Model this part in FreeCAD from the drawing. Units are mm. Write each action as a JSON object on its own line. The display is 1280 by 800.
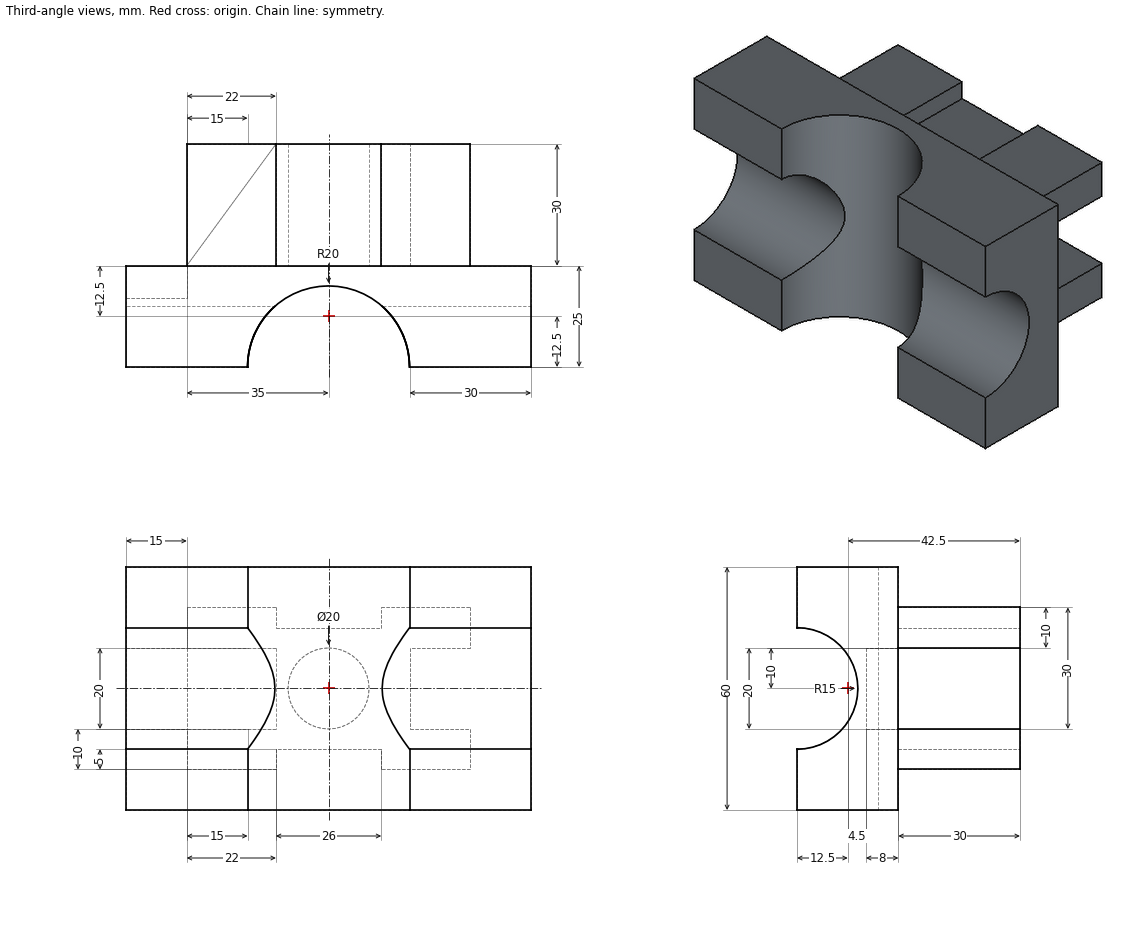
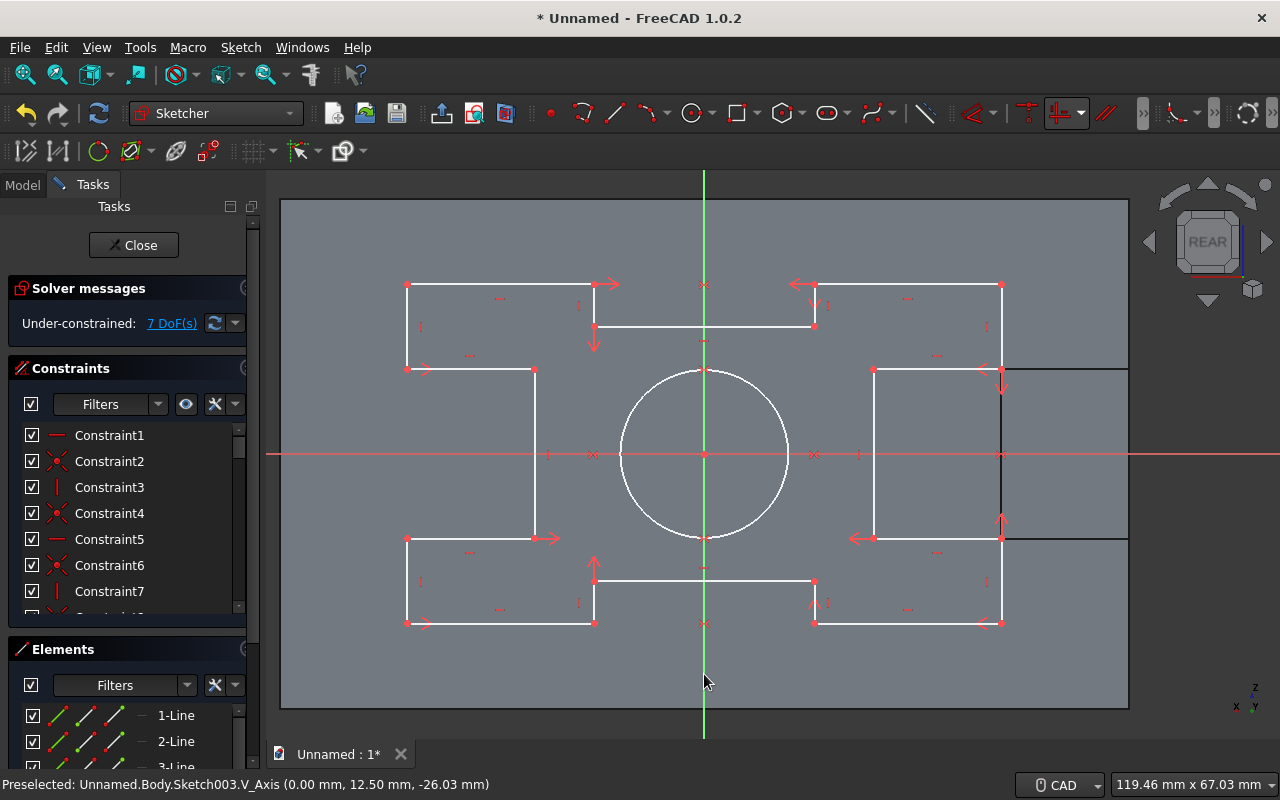
{"action": "left_click", "coordinate": [972, 114]}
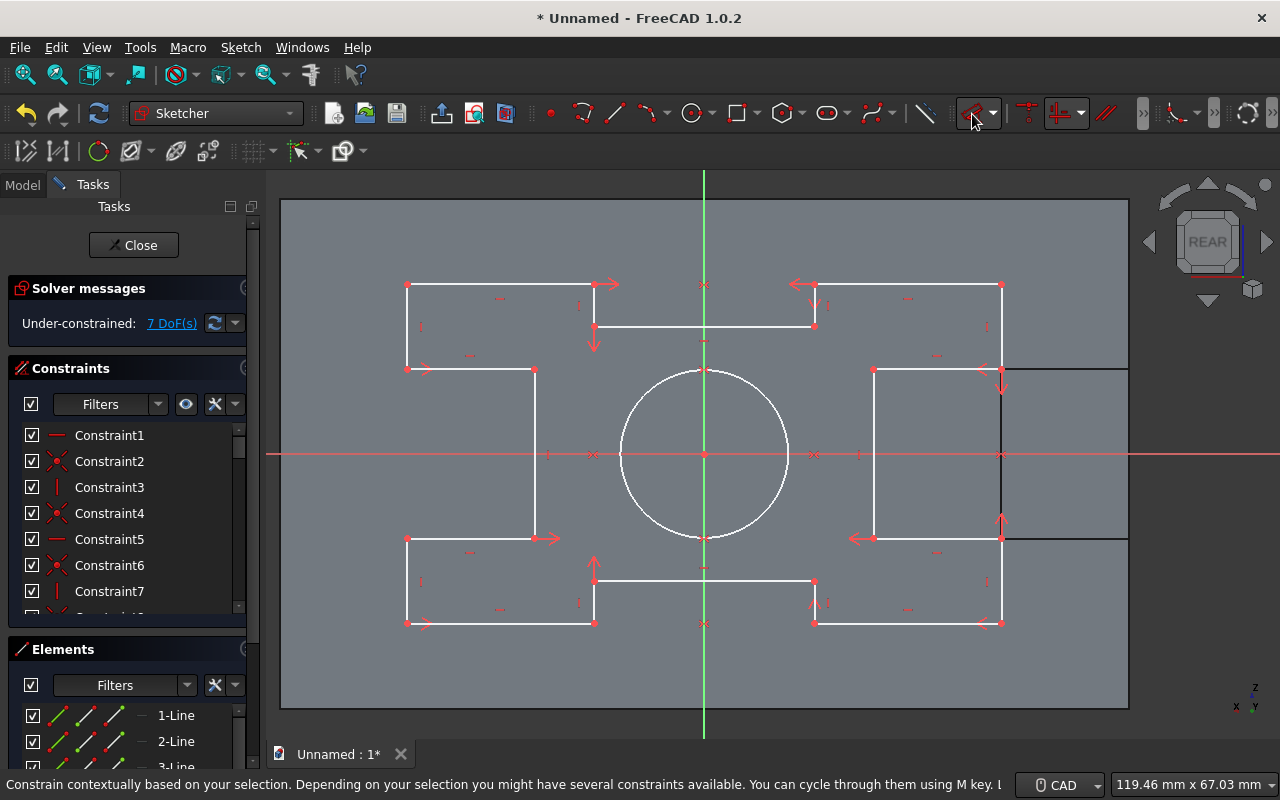
{"action": "left_click", "coordinate": [763, 394]}
{"action": "left_click", "coordinate": [785, 371]}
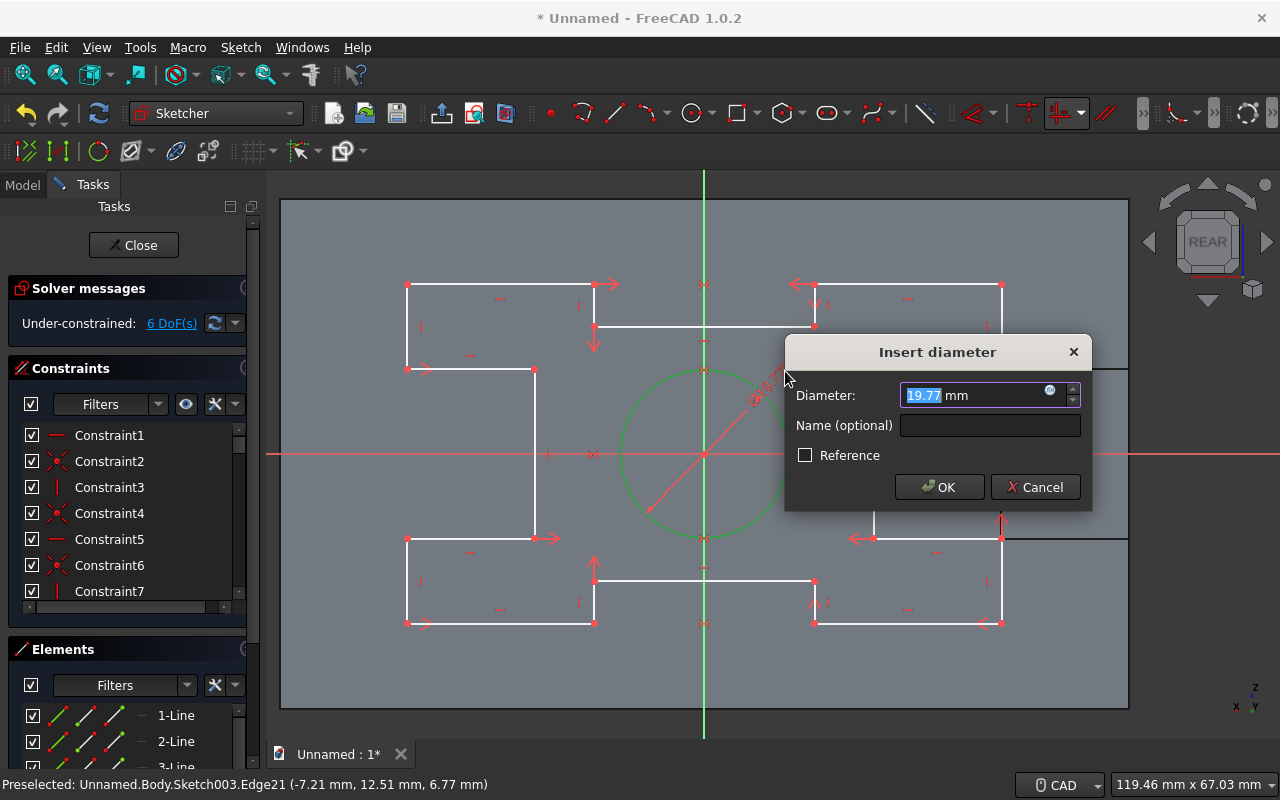
{"action": "type", "text": "20"}
{"action": "key", "text": "Return"}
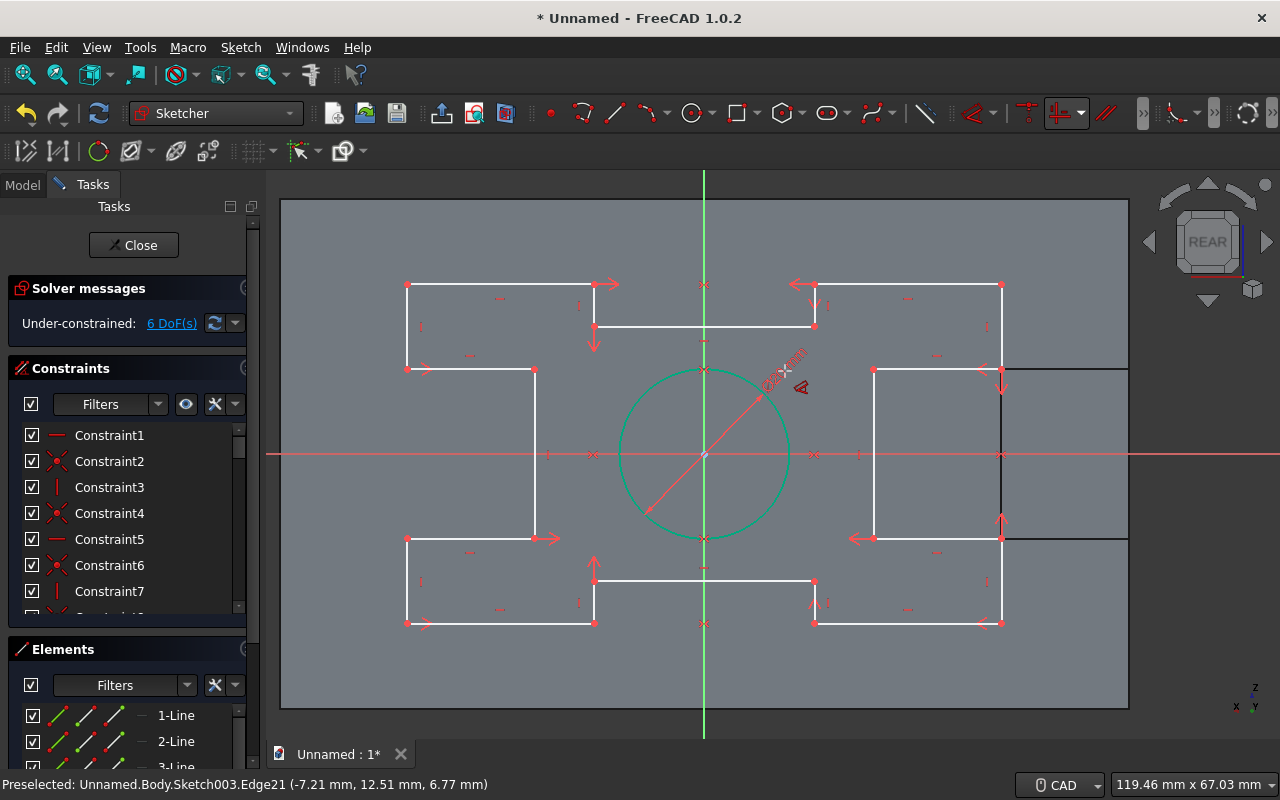
{"action": "left_click", "coordinate": [815, 594]}
{"action": "left_click", "coordinate": [849, 603]}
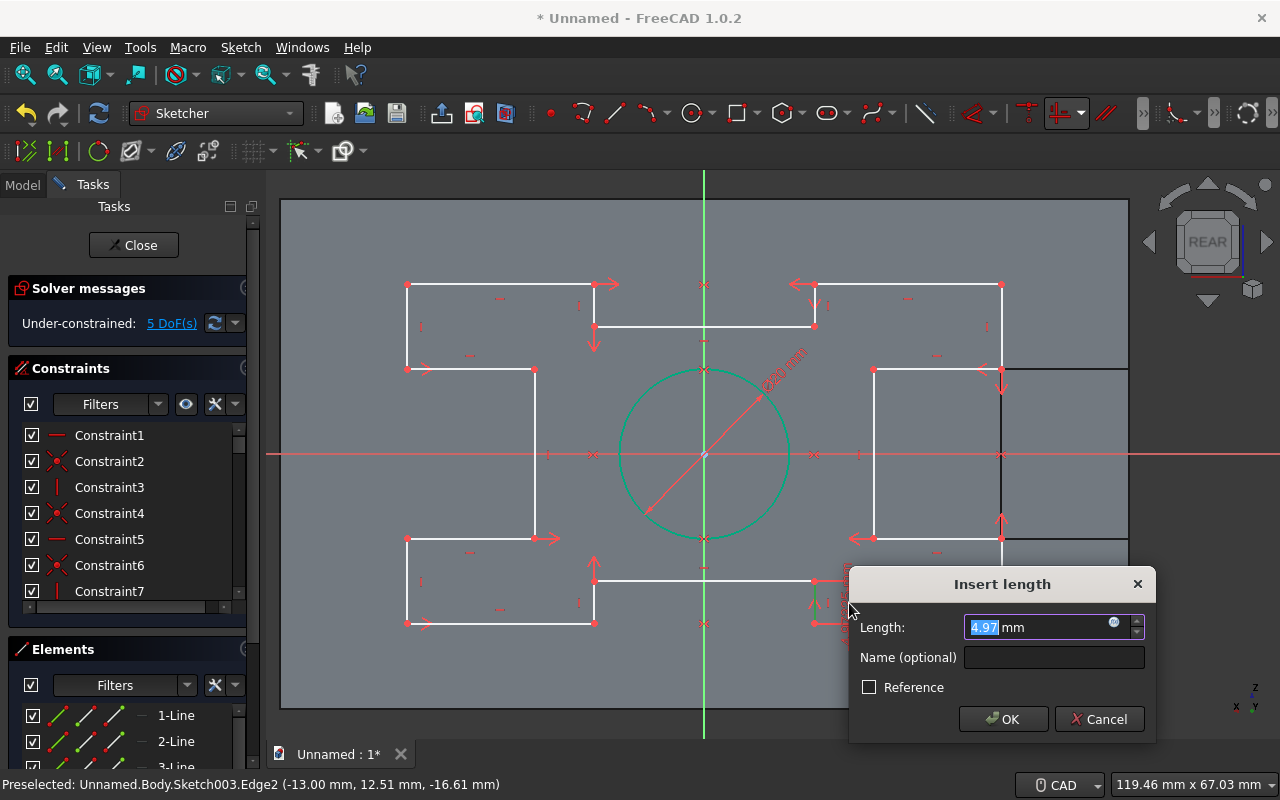
{"action": "type", "text": "5"}
{"action": "key", "text": "Return"}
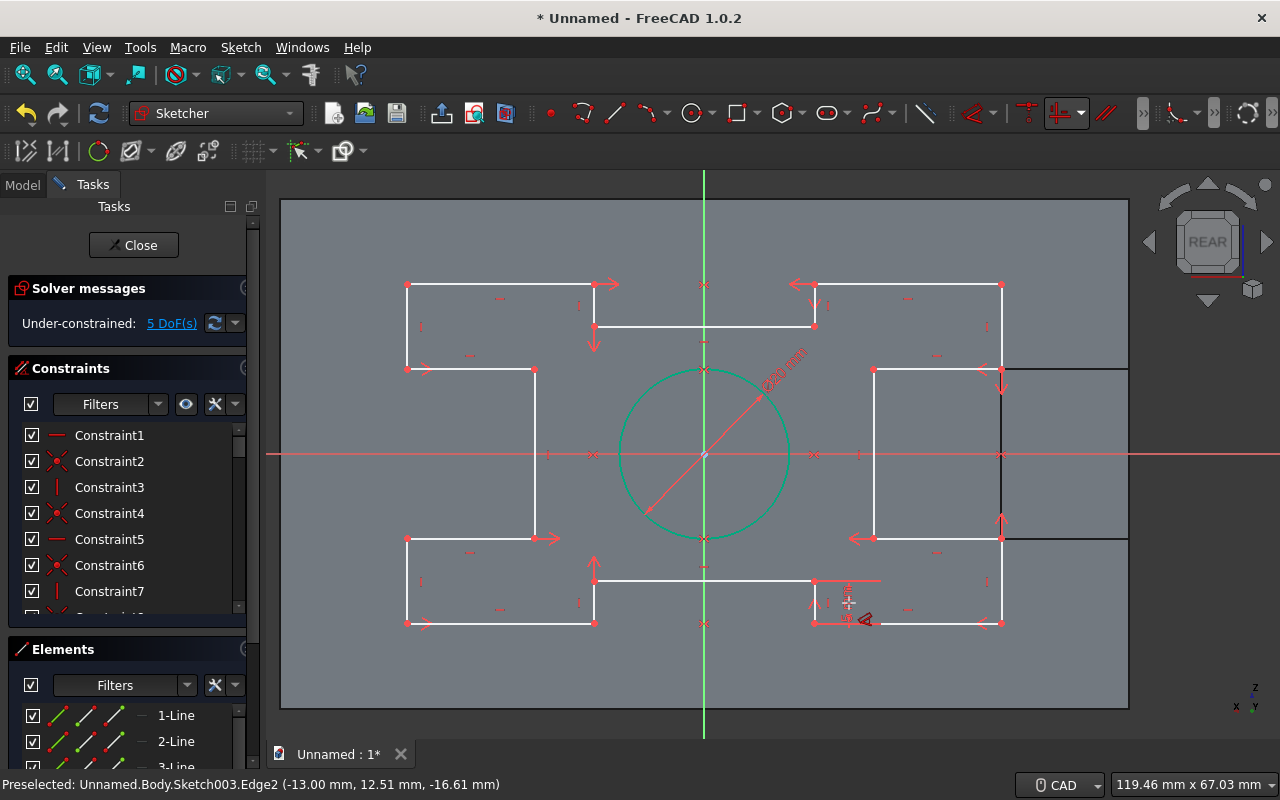
{"action": "left_click", "coordinate": [660, 581]}
{"action": "left_click", "coordinate": [654, 615]}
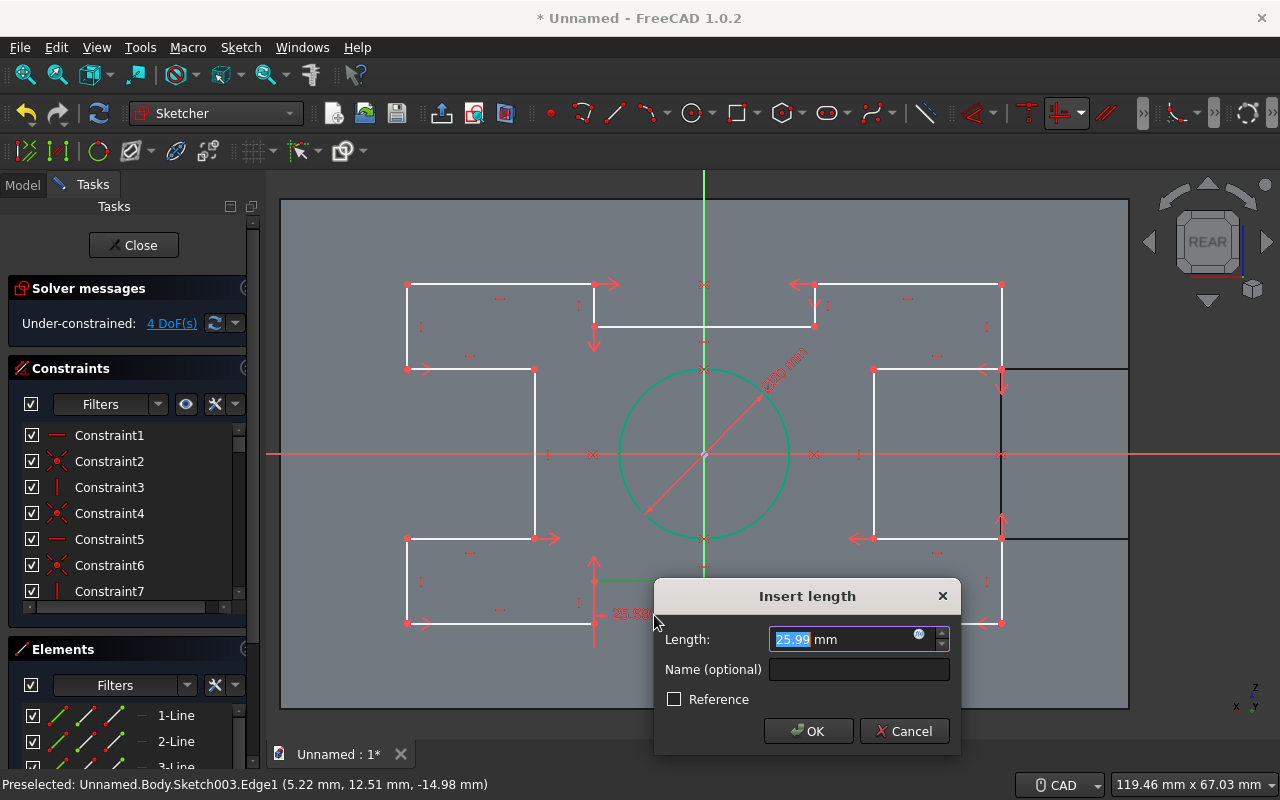
{"action": "type", "text": "26"}
{"action": "key", "text": "Return"}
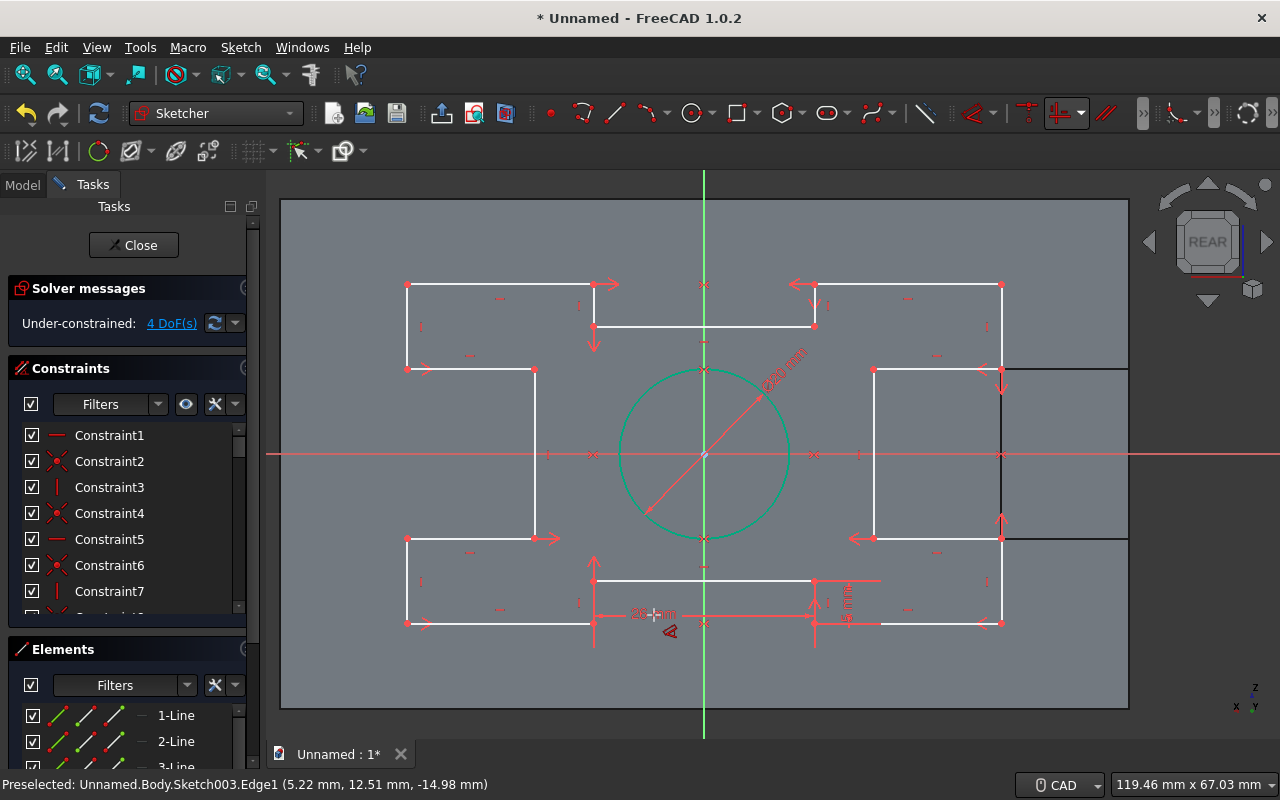
{"action": "left_click", "coordinate": [871, 624]}
{"action": "left_click", "coordinate": [908, 658]}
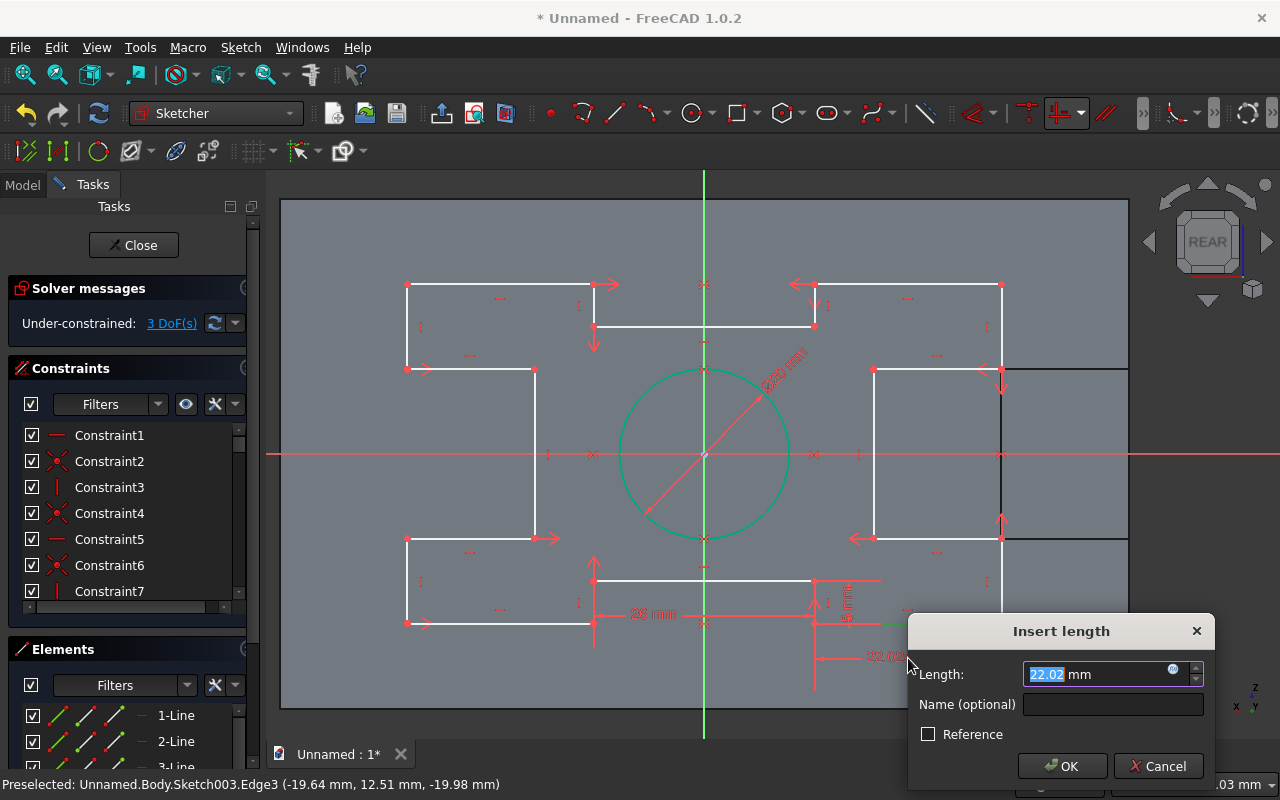
{"action": "type", "text": "22"}
{"action": "key", "text": "Return"}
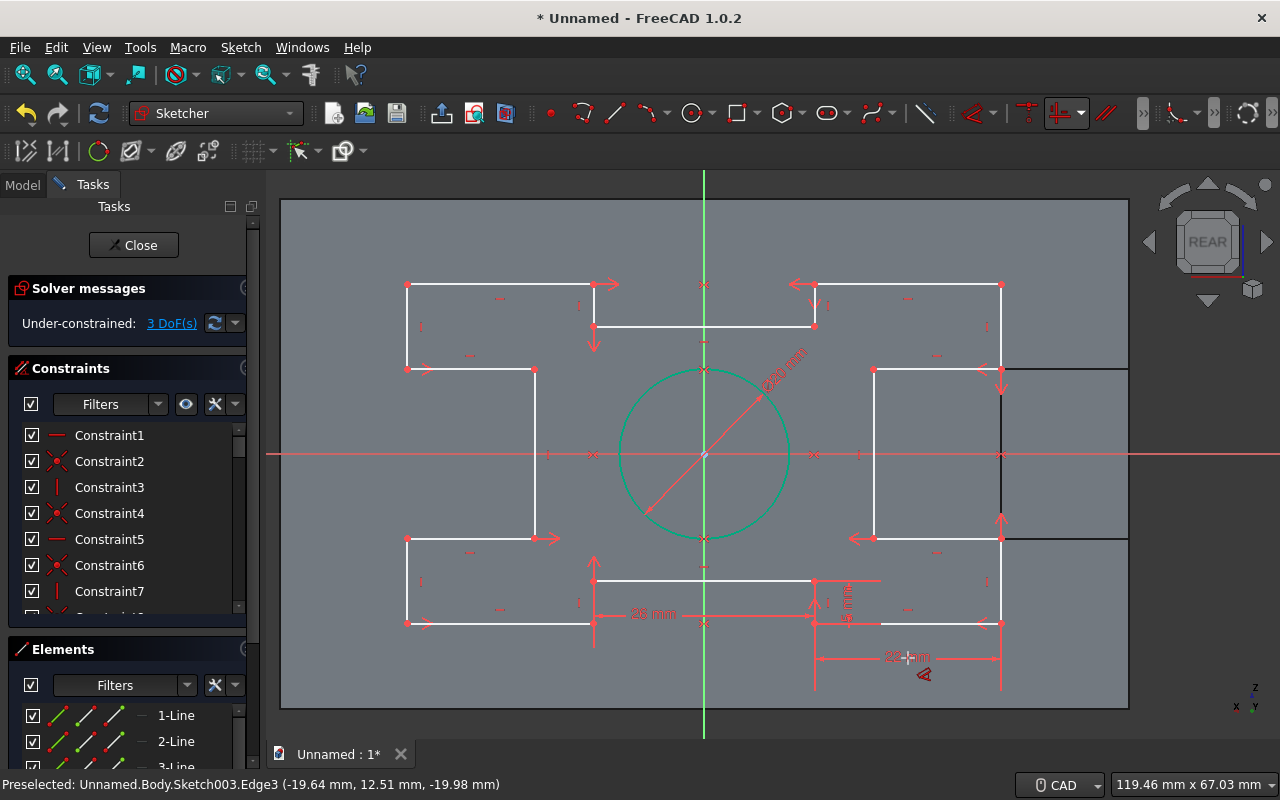
{"action": "left_click", "coordinate": [1001, 598]}
{"action": "left_click", "coordinate": [1035, 581]}